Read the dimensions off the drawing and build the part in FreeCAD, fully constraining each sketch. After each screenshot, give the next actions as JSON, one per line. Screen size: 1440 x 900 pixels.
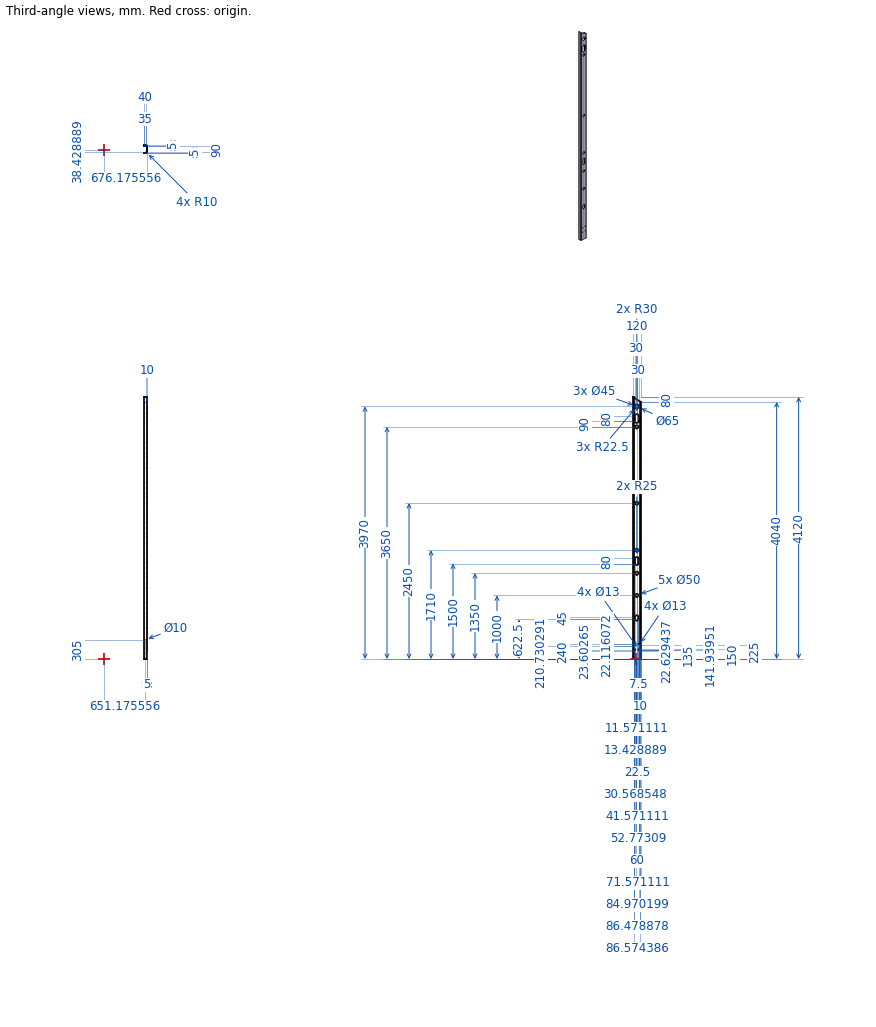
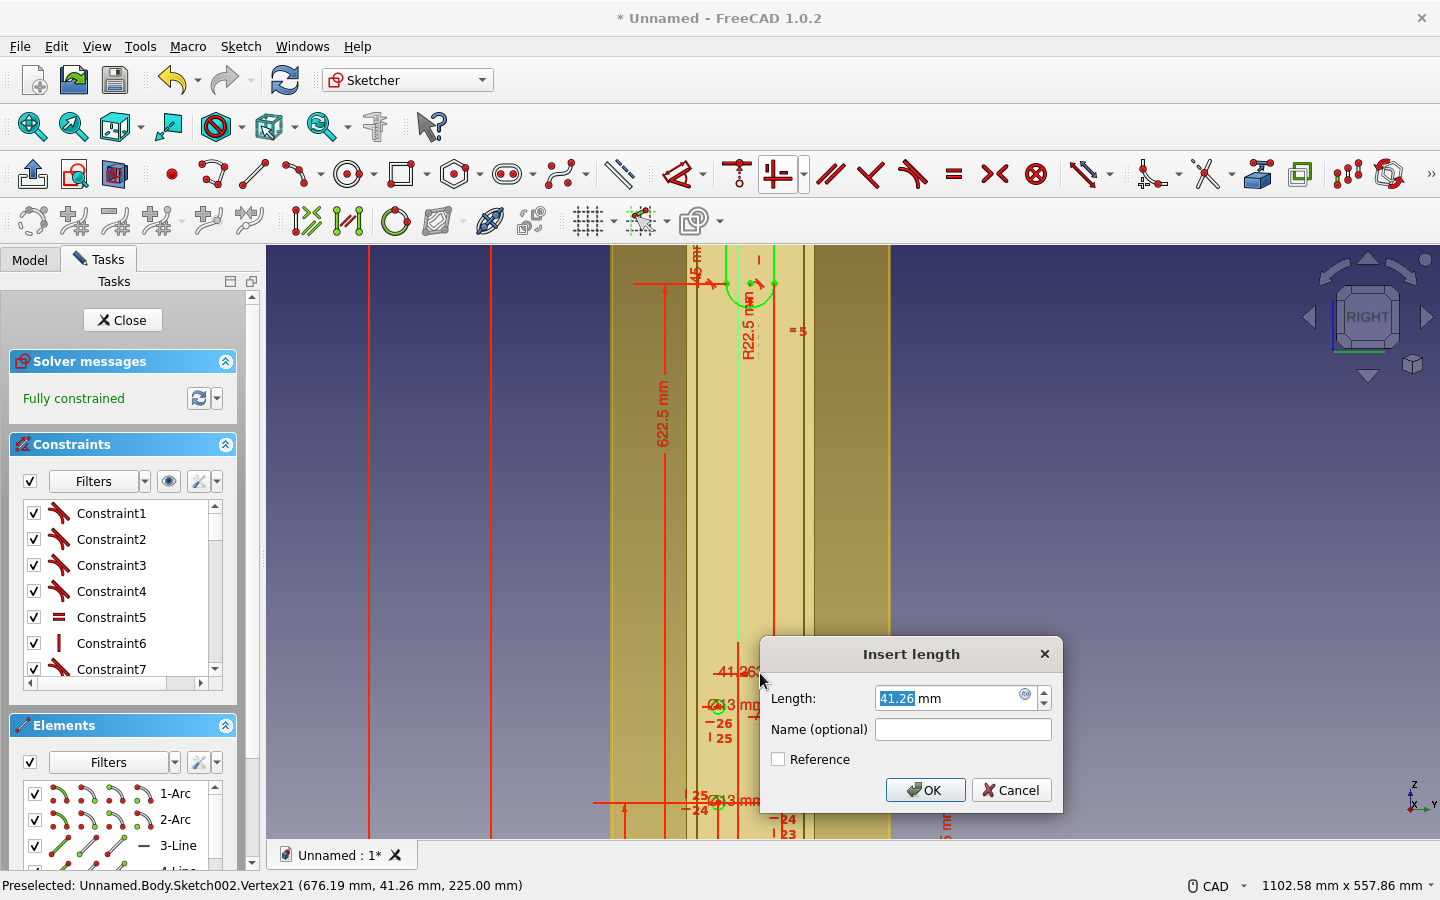
{"action": "type", "text": "41.571111"}
{"action": "key", "text": "Return"}
{"action": "key", "text": "Escape"}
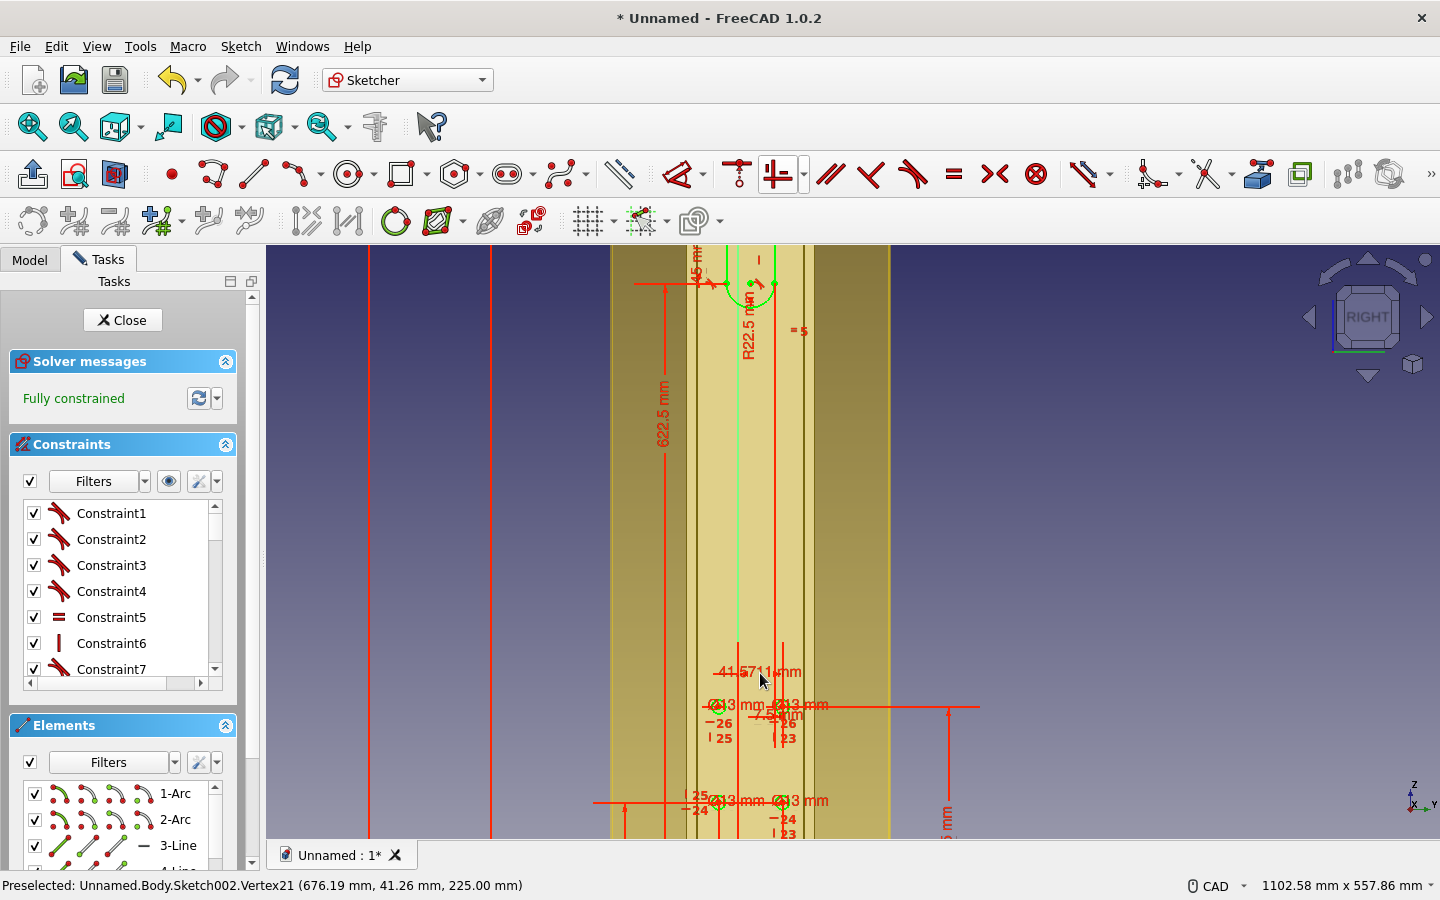
{"action": "left_click", "coordinate": [123, 320]}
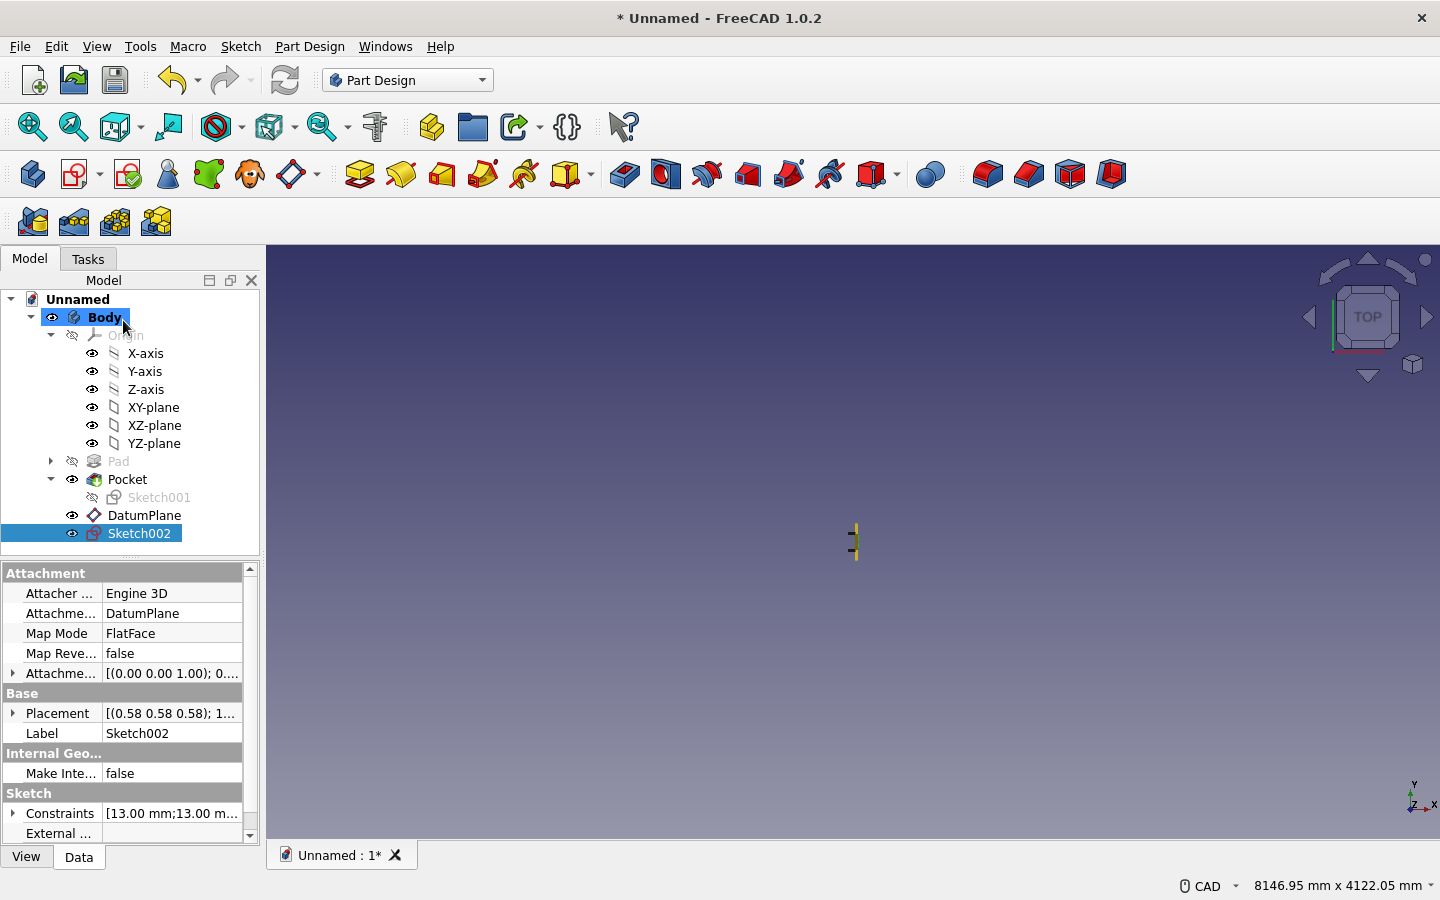
{"action": "left_click", "coordinate": [625, 174]}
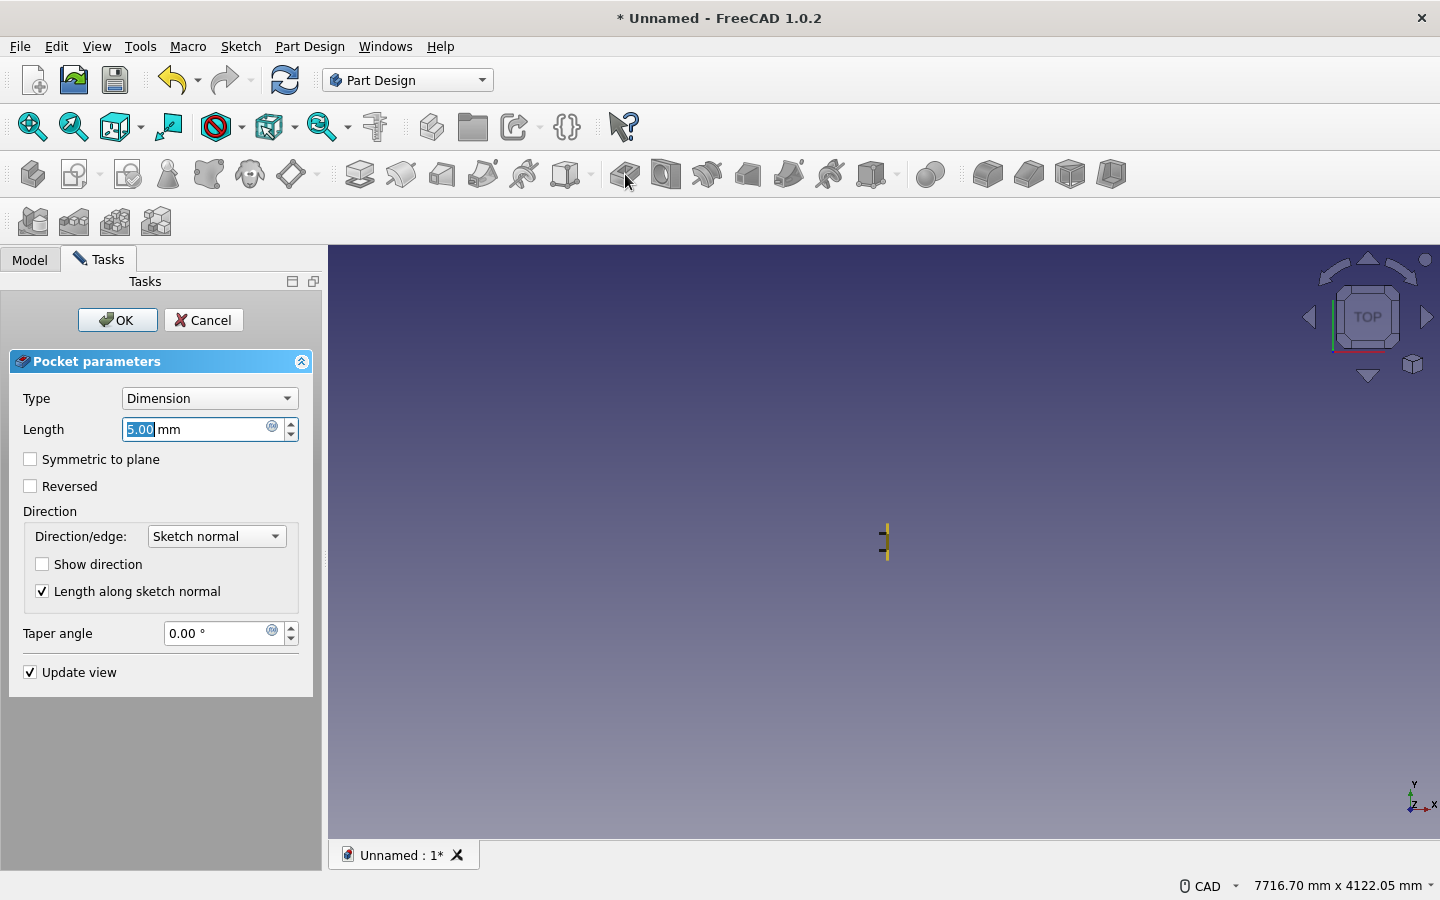
{"action": "type", "text": "10"}
{"action": "key", "text": "Tab"}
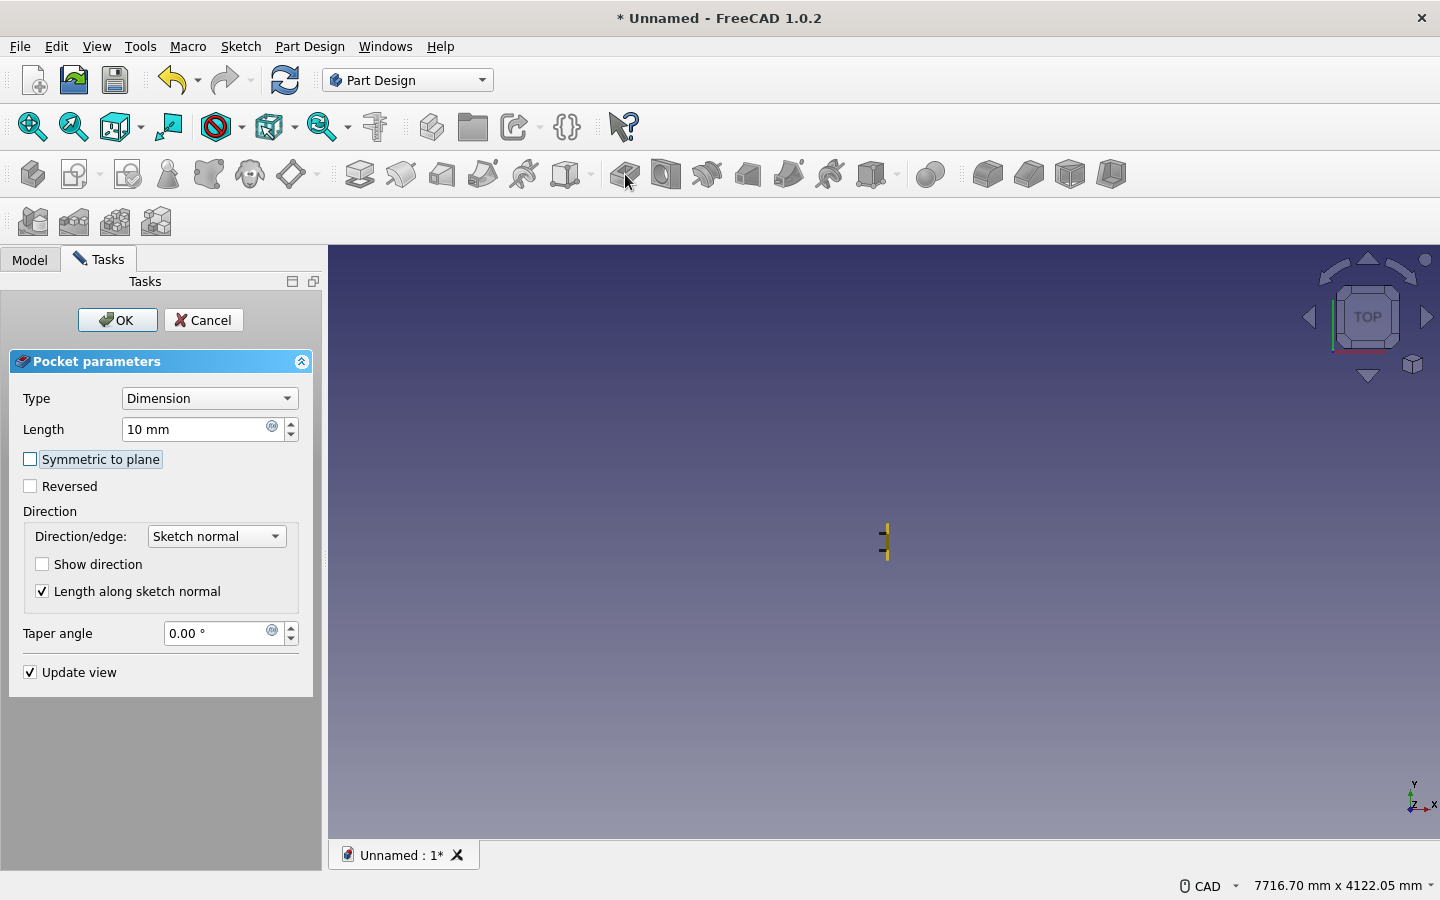
{"action": "left_click", "coordinate": [118, 320]}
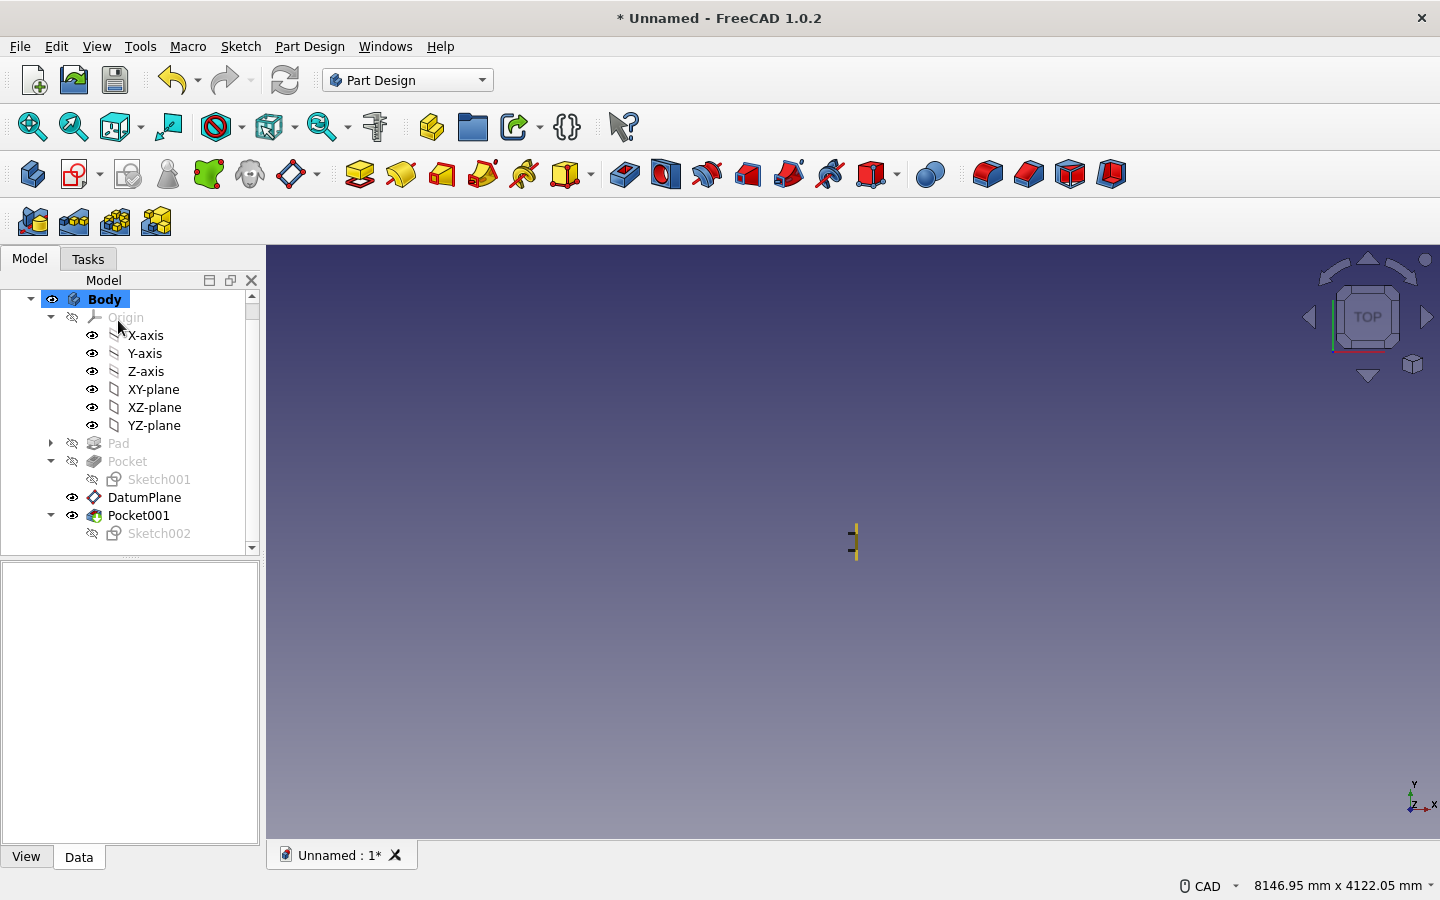
{"action": "left_click", "coordinate": [117, 497]}
{"action": "key", "text": "space"}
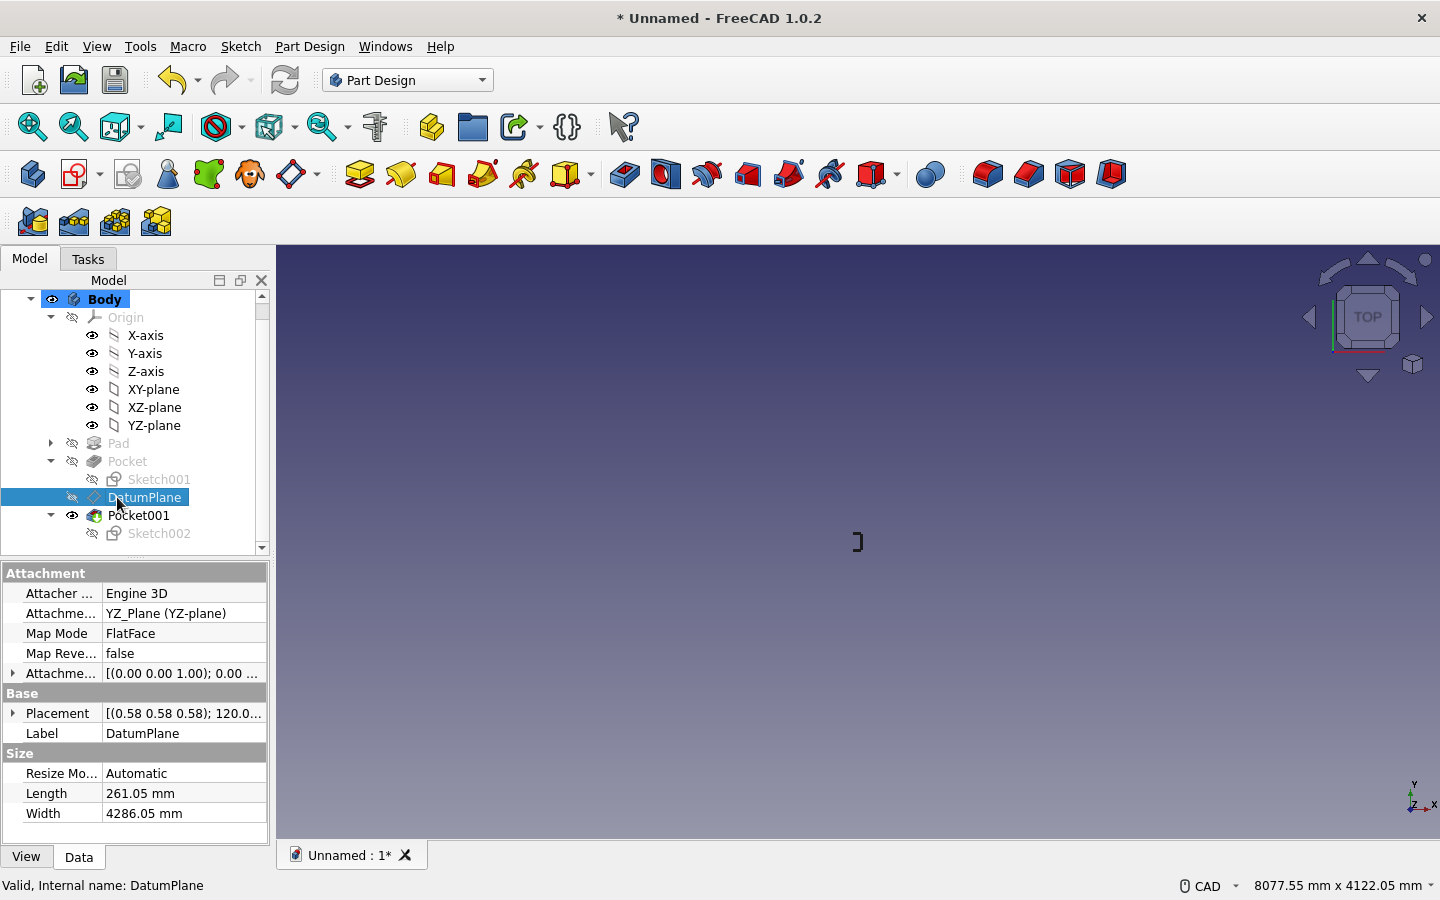
{"action": "key", "text": "v f"}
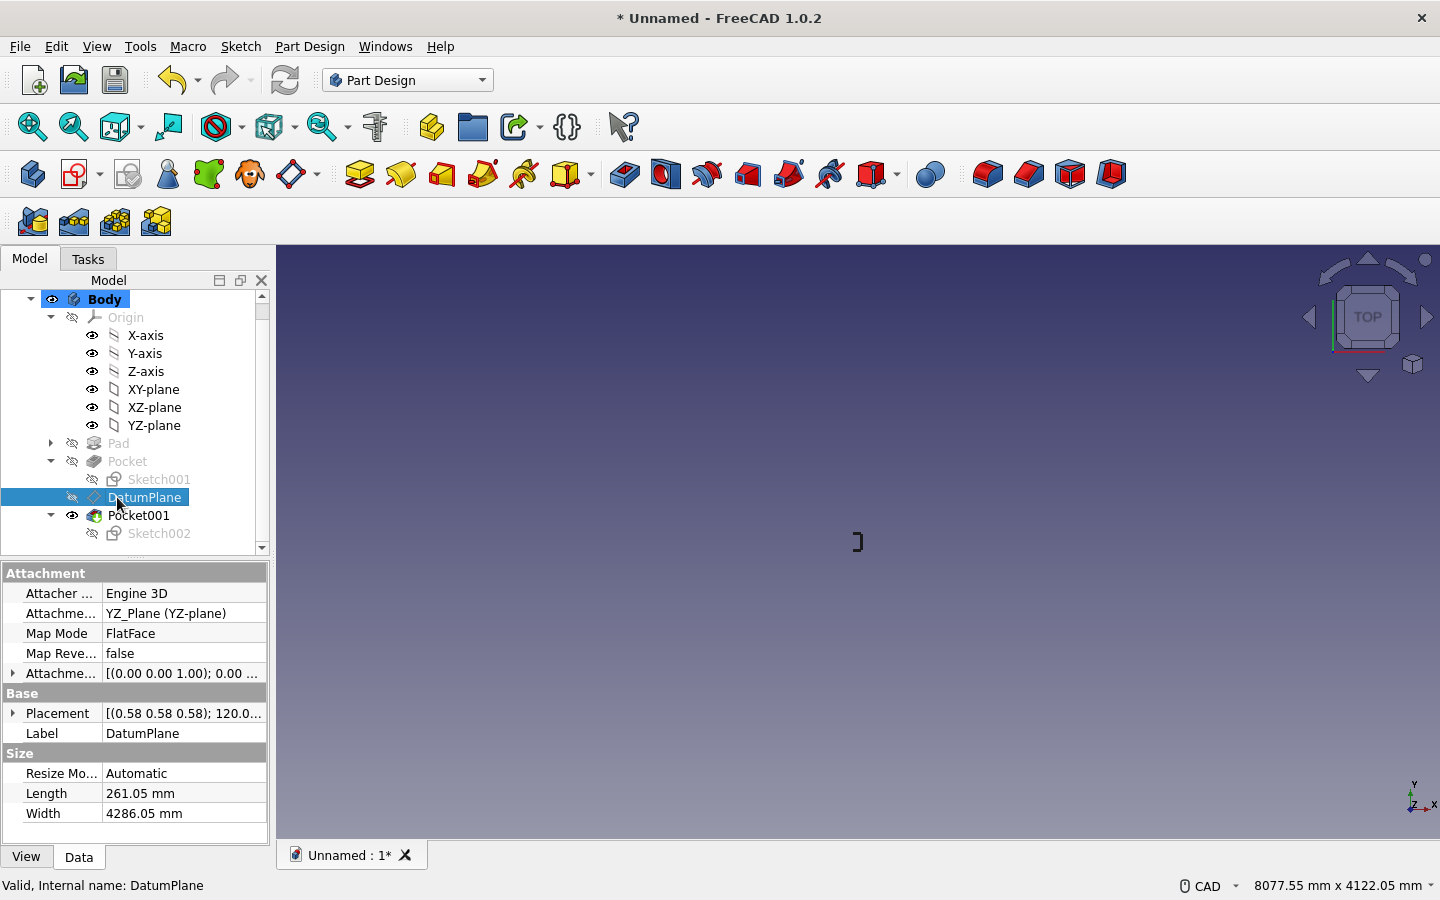
{"action": "key", "text": "0"}